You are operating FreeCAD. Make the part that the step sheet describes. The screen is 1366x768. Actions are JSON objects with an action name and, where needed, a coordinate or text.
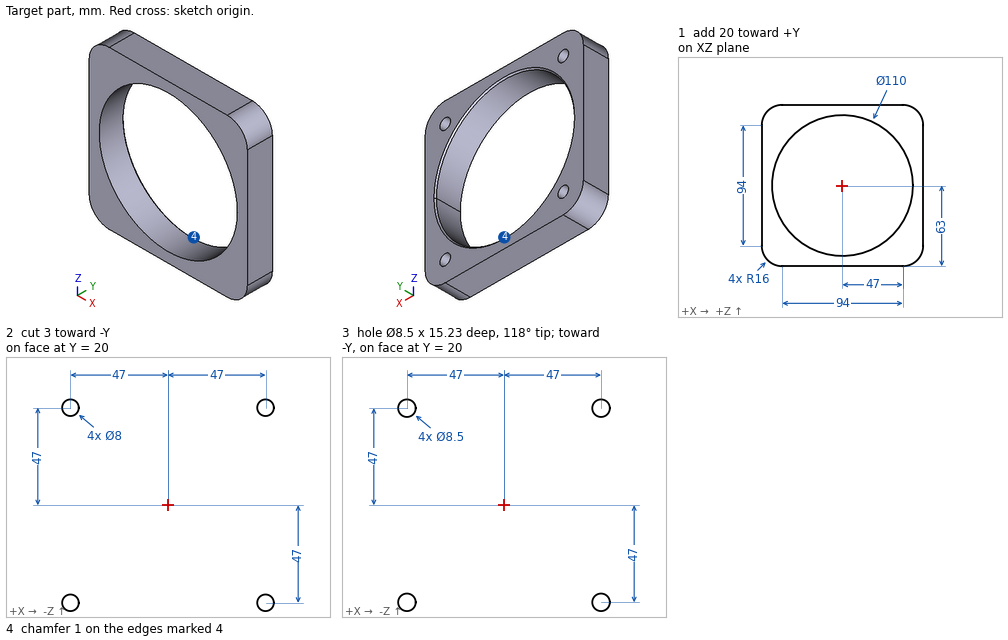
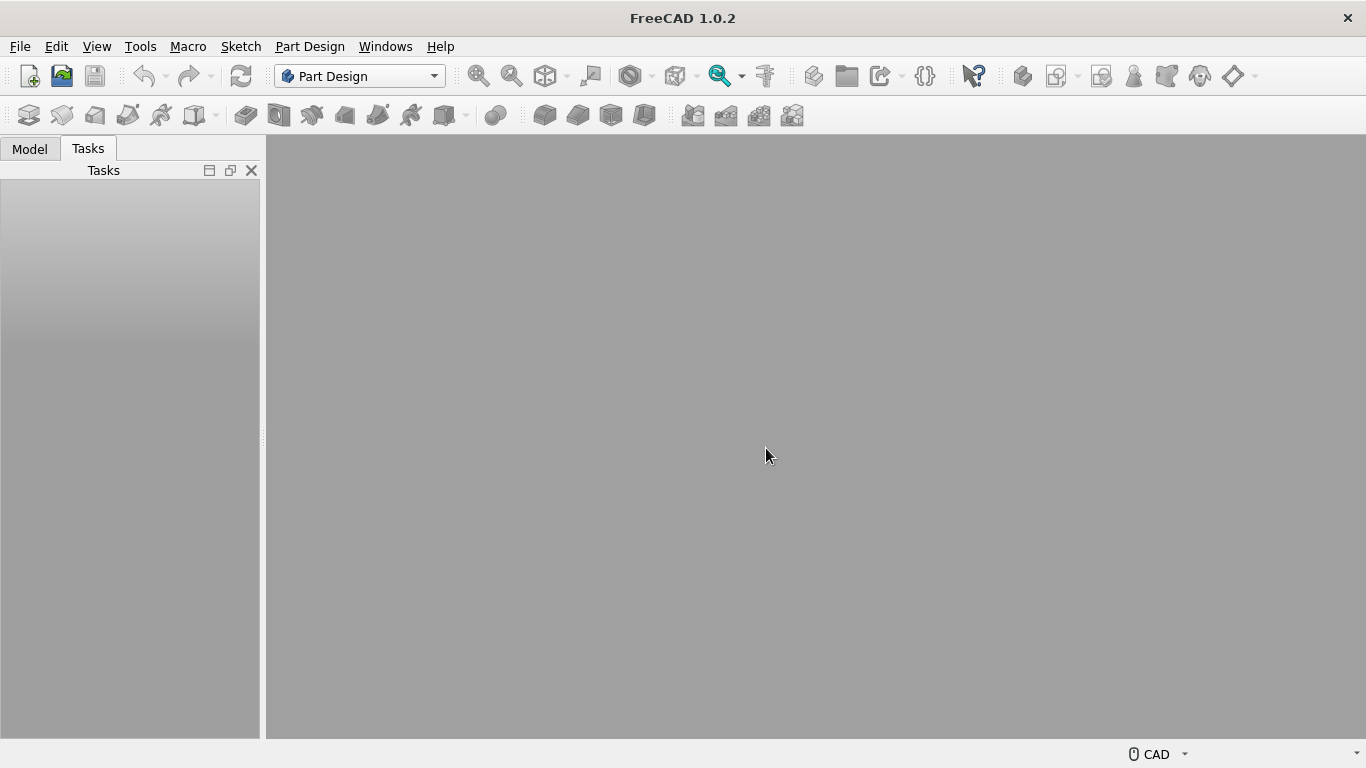
{"action": "left_click", "coordinate": [29, 76]}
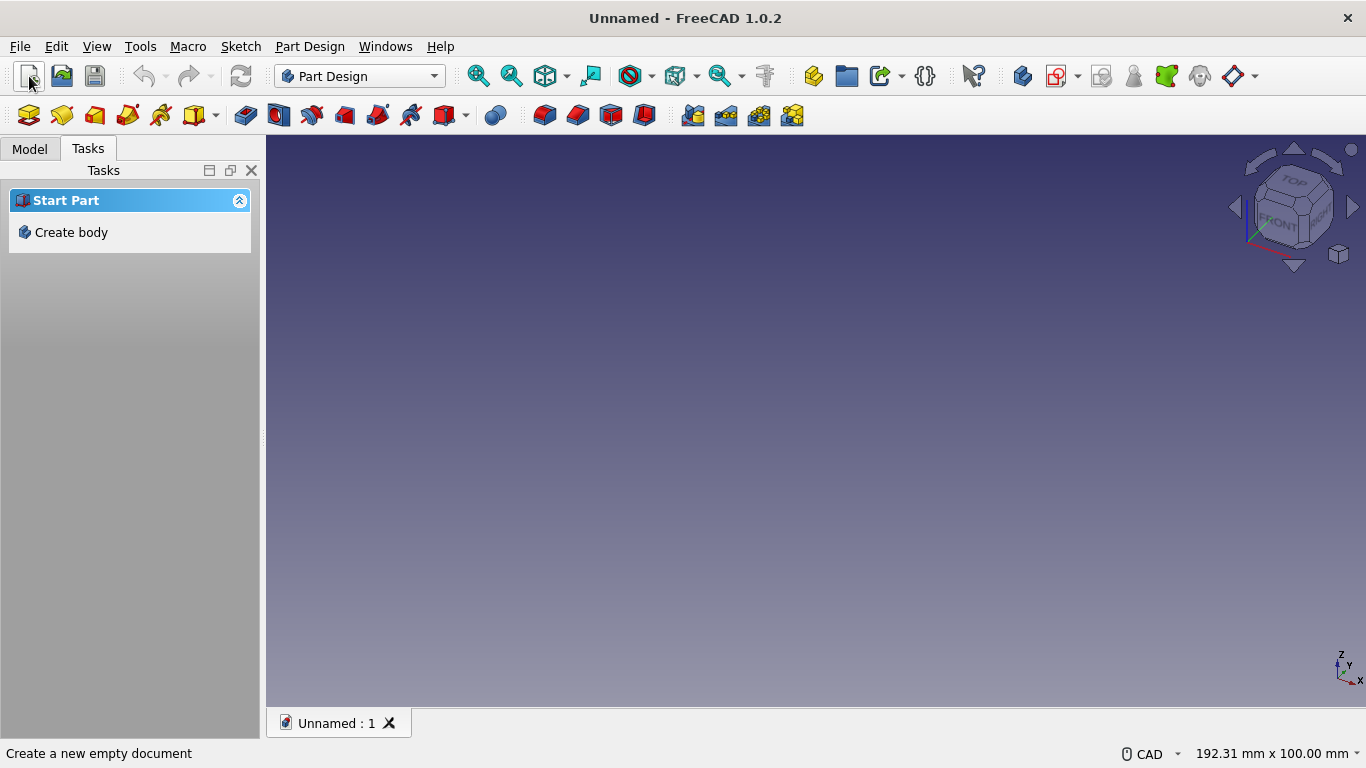
{"action": "left_click", "coordinate": [1056, 76]}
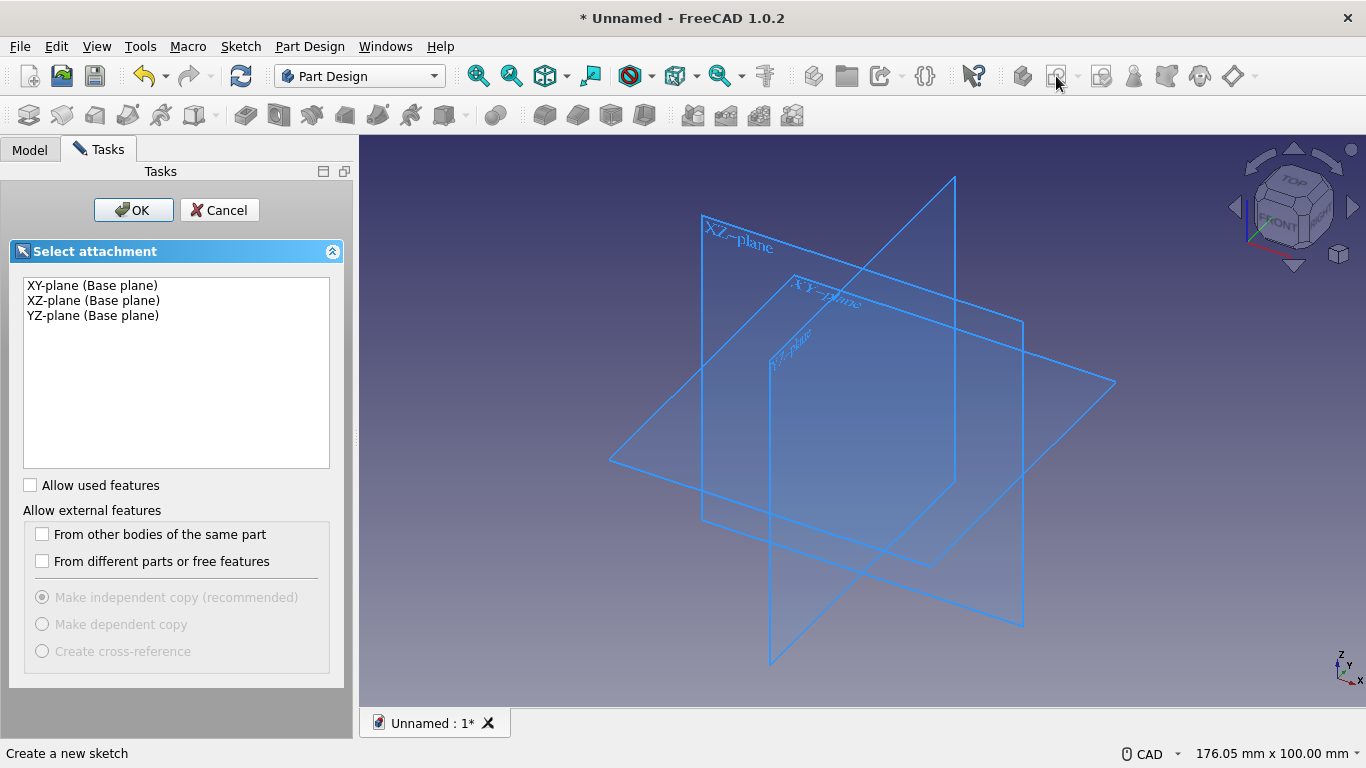
{"action": "left_click", "coordinate": [84, 300]}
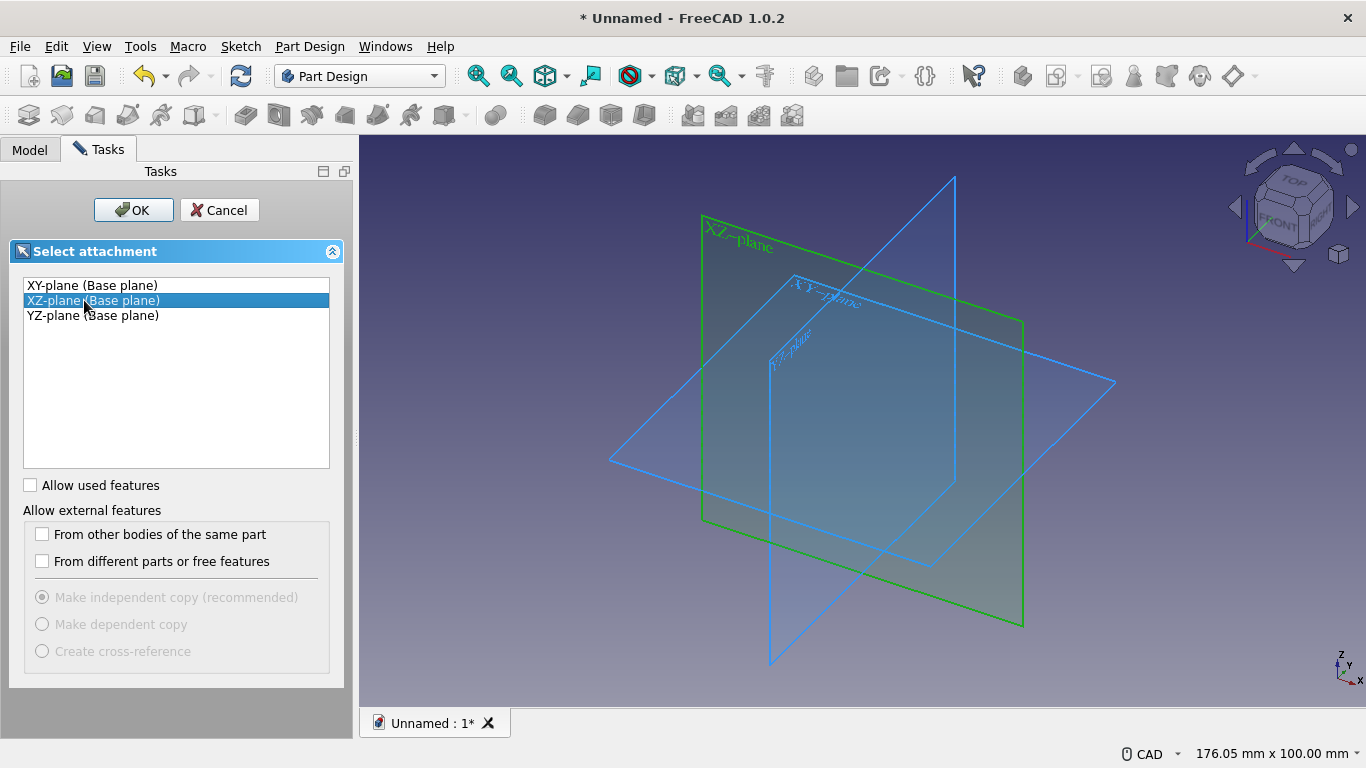
{"action": "left_click", "coordinate": [134, 210]}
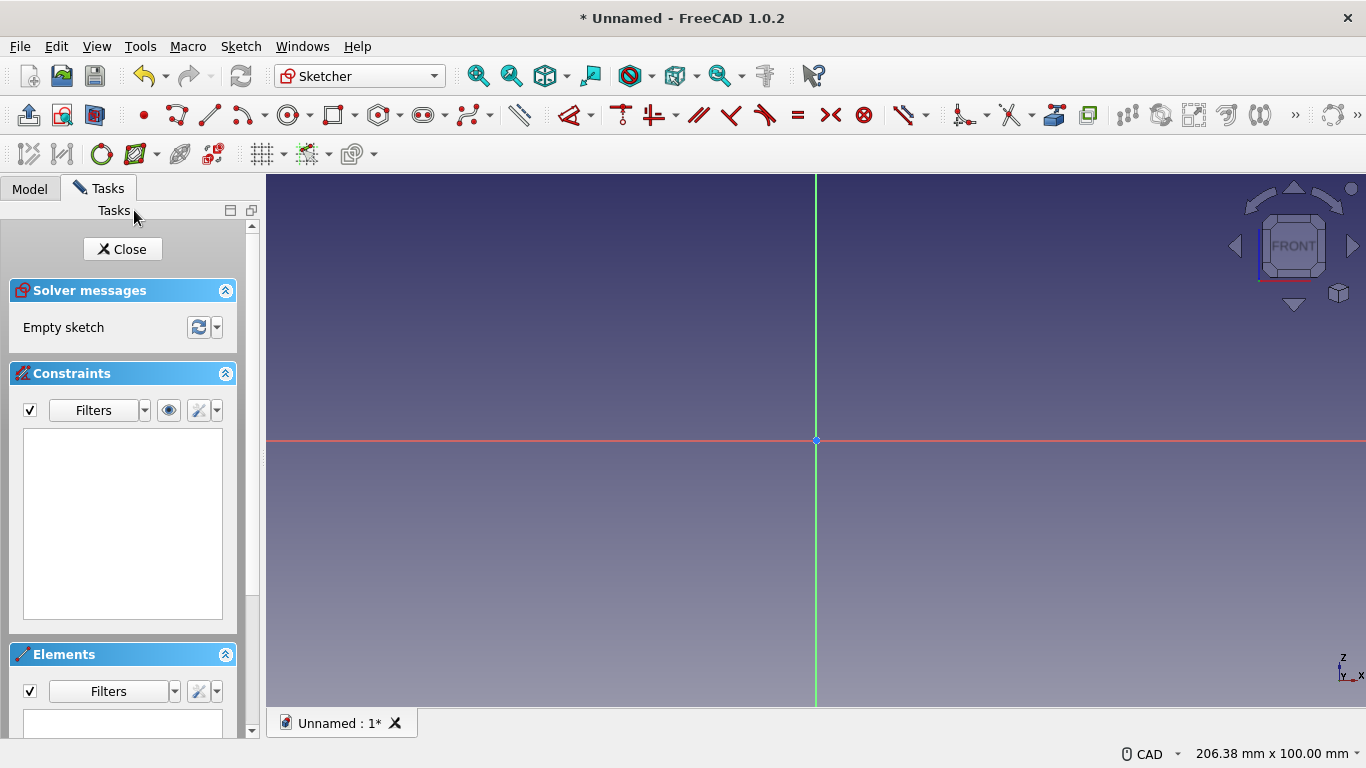
{"action": "scroll", "coordinate": [664, 440], "scroll_direction": "down", "scroll_amount": 3}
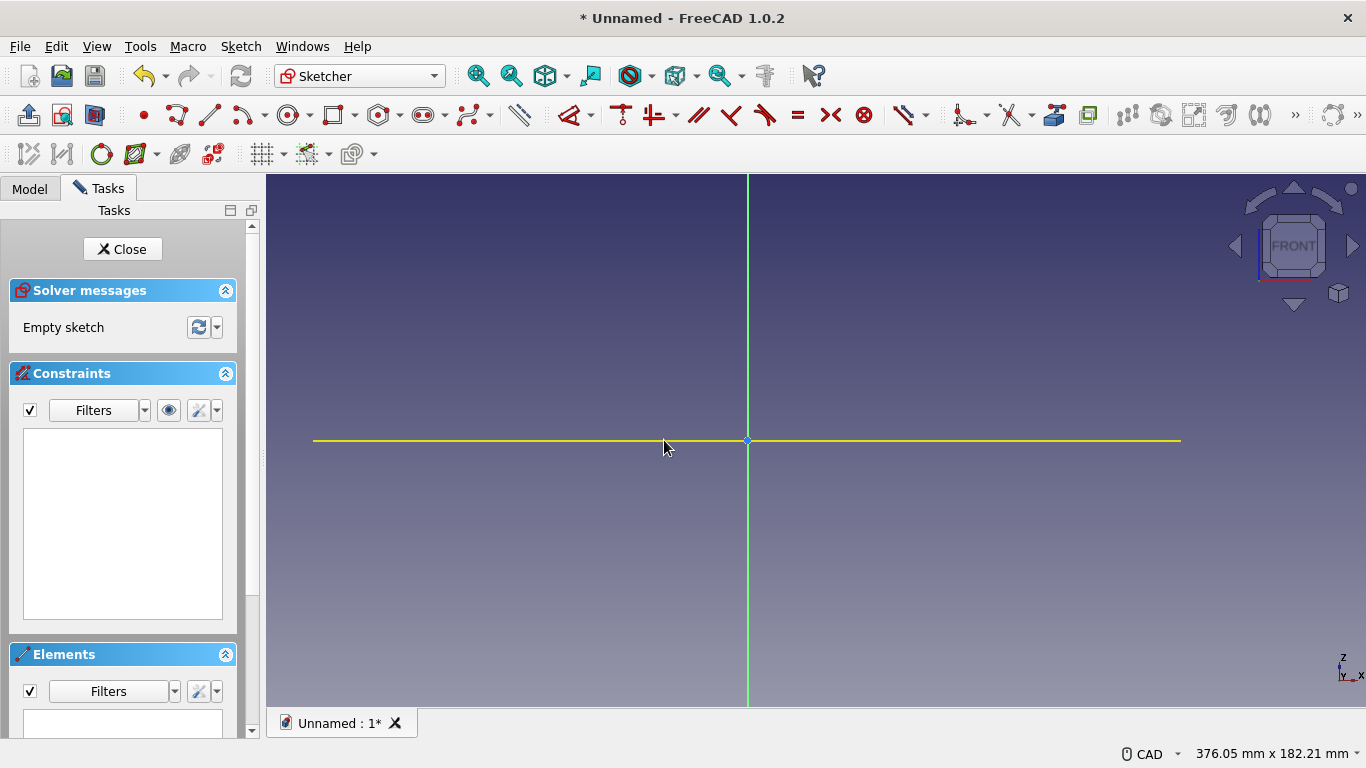
{"action": "key", "text": "g l"}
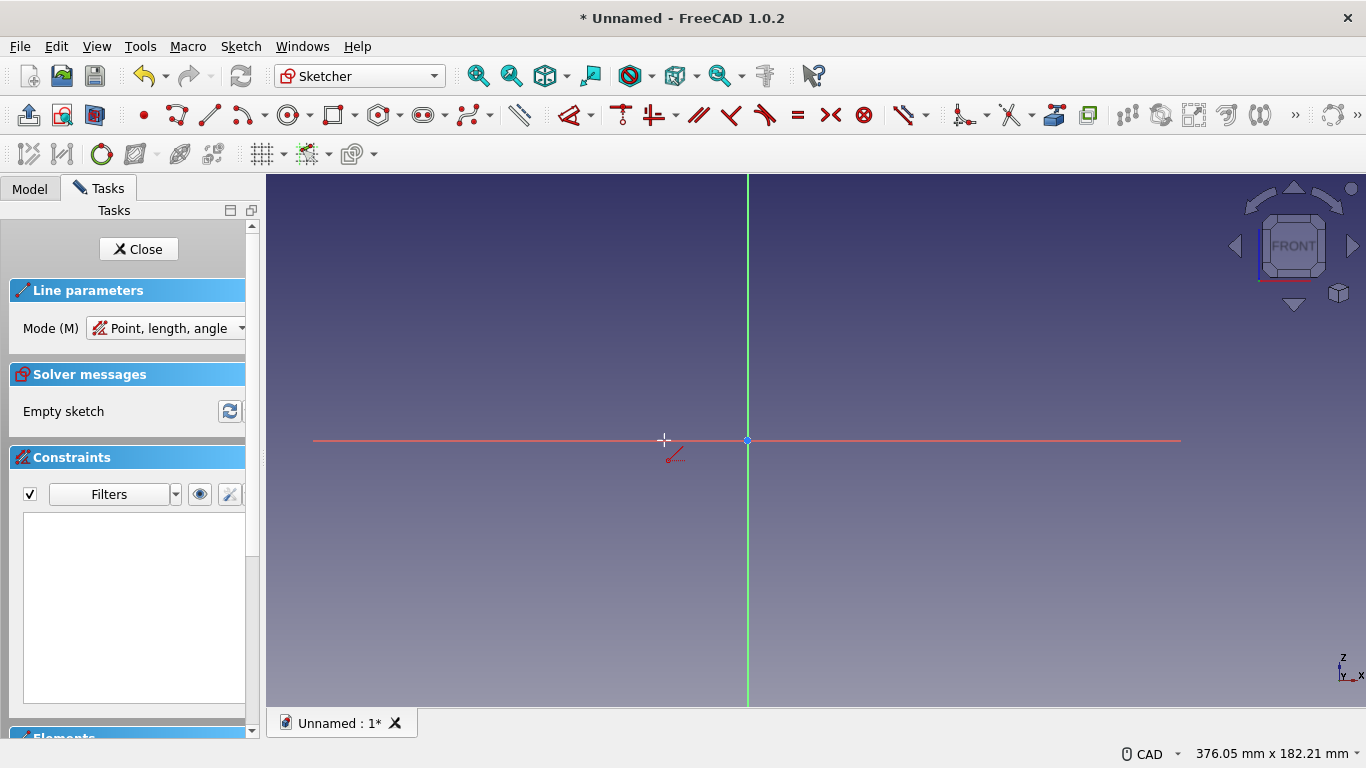
{"action": "left_click", "coordinate": [885, 625]}
{"action": "left_click", "coordinate": [610, 625]}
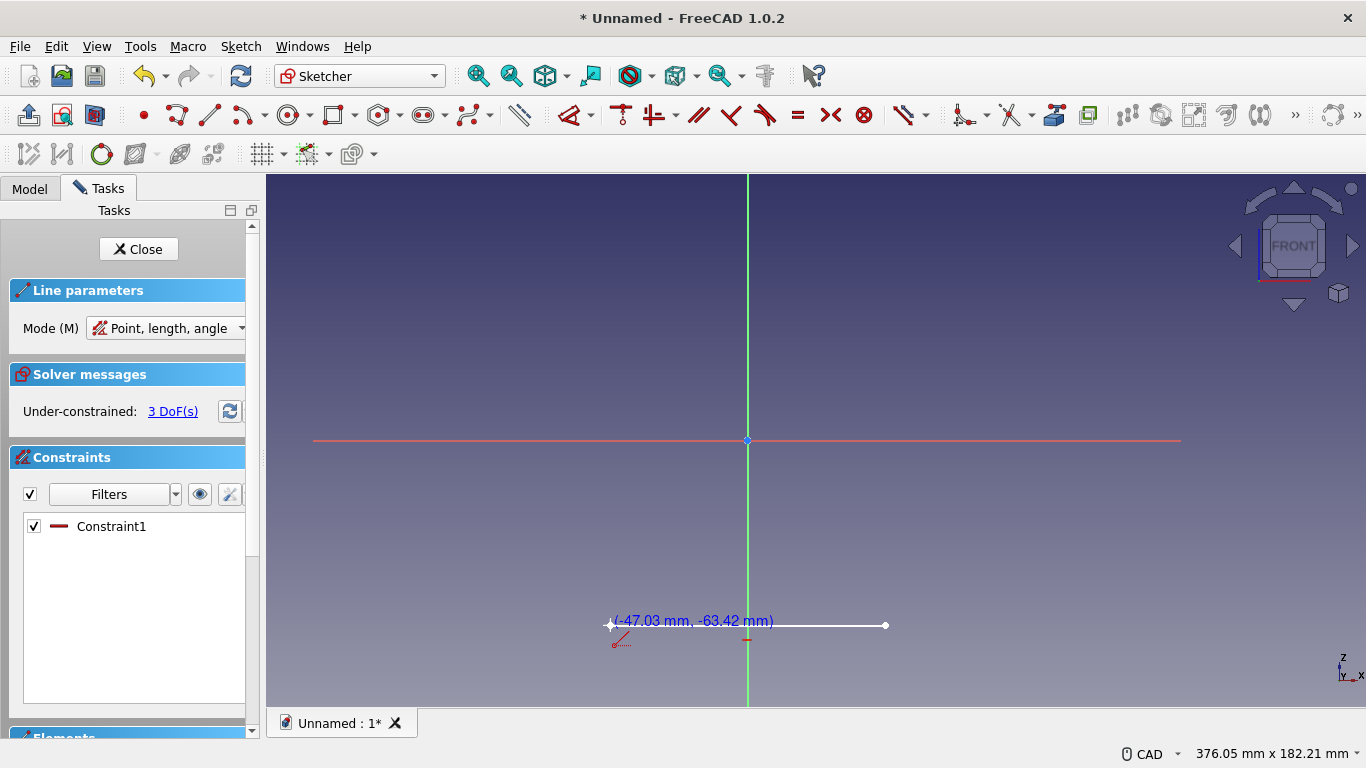
{"action": "left_click", "coordinate": [563, 578]}
{"action": "left_click", "coordinate": [563, 303]}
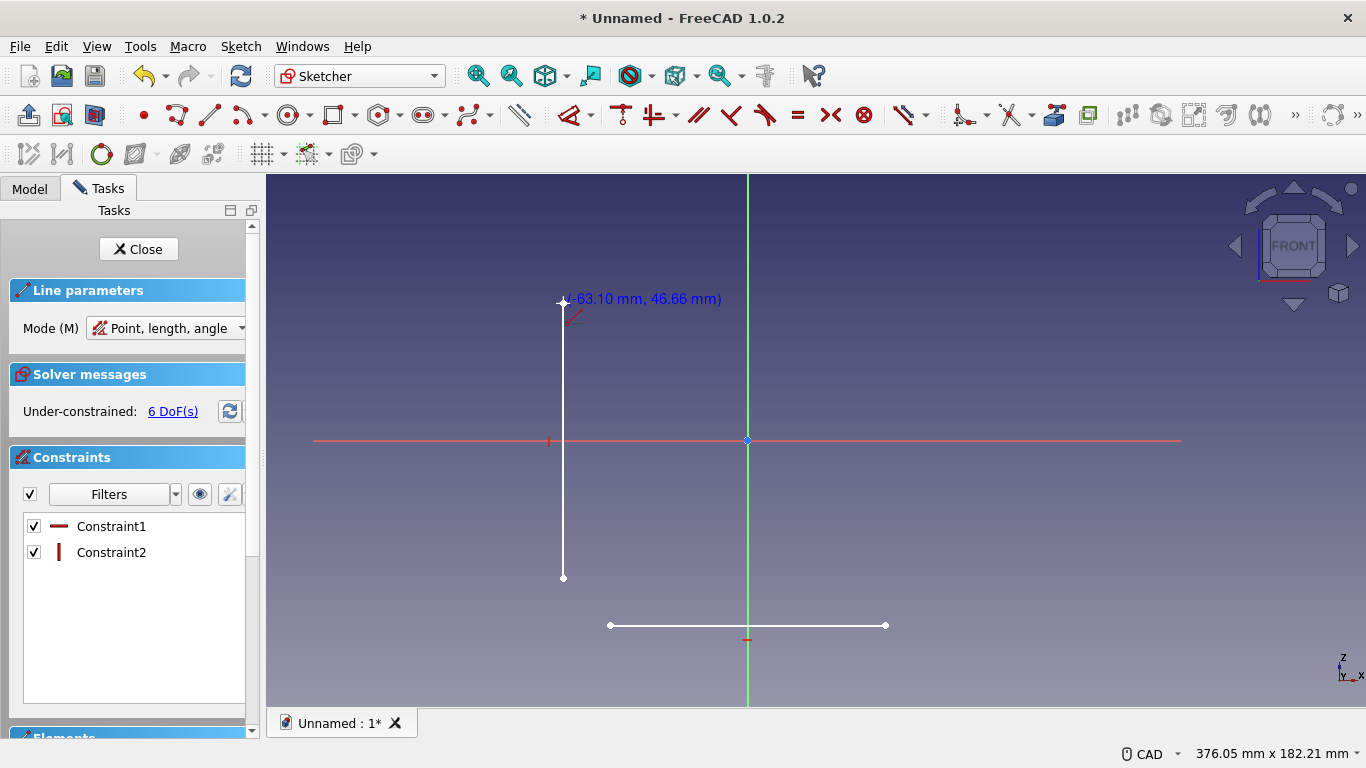
{"action": "left_click", "coordinate": [610, 256]}
{"action": "left_click", "coordinate": [885, 256]}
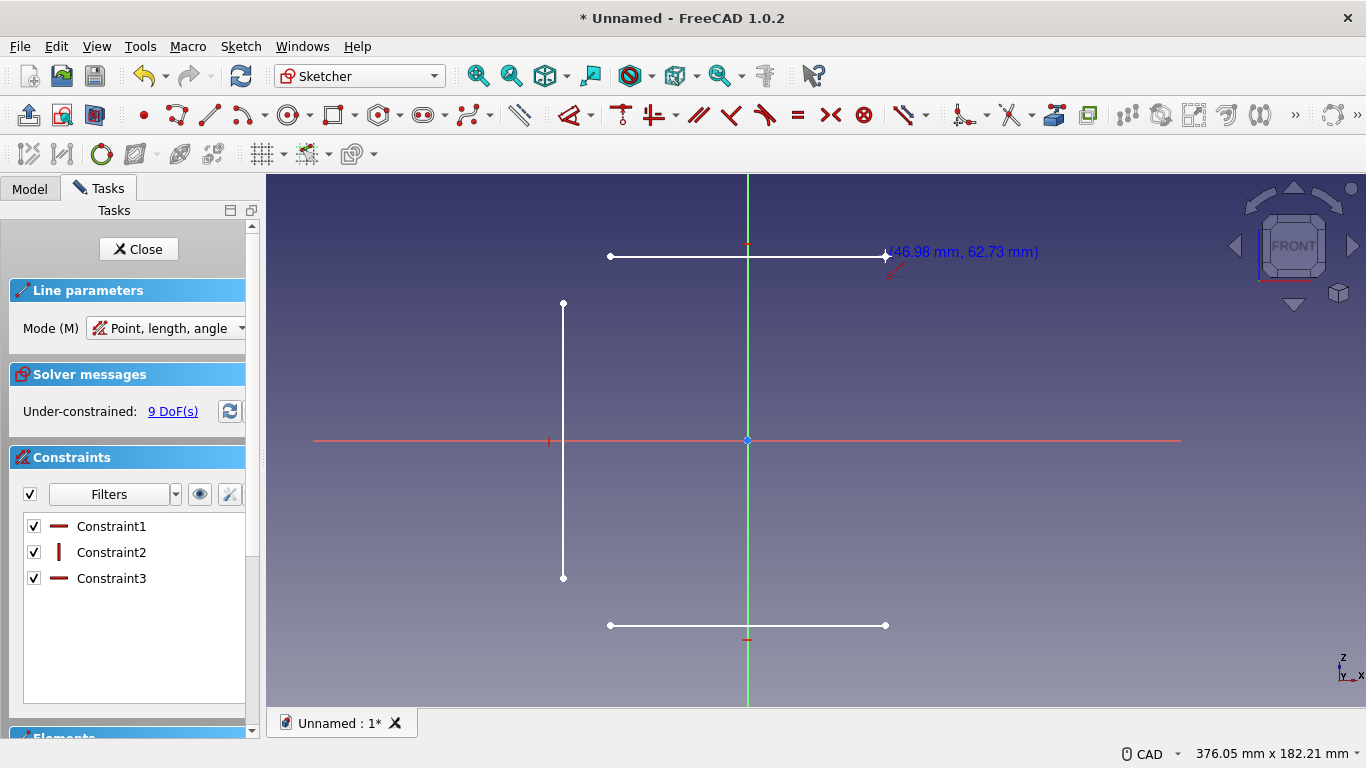
{"action": "left_click", "coordinate": [932, 303]}
{"action": "left_click", "coordinate": [932, 578]}